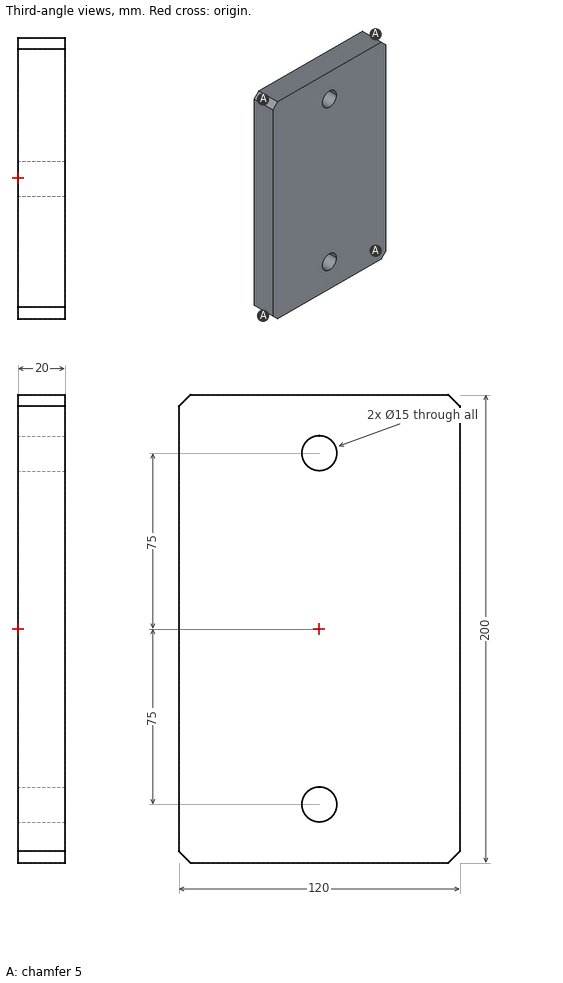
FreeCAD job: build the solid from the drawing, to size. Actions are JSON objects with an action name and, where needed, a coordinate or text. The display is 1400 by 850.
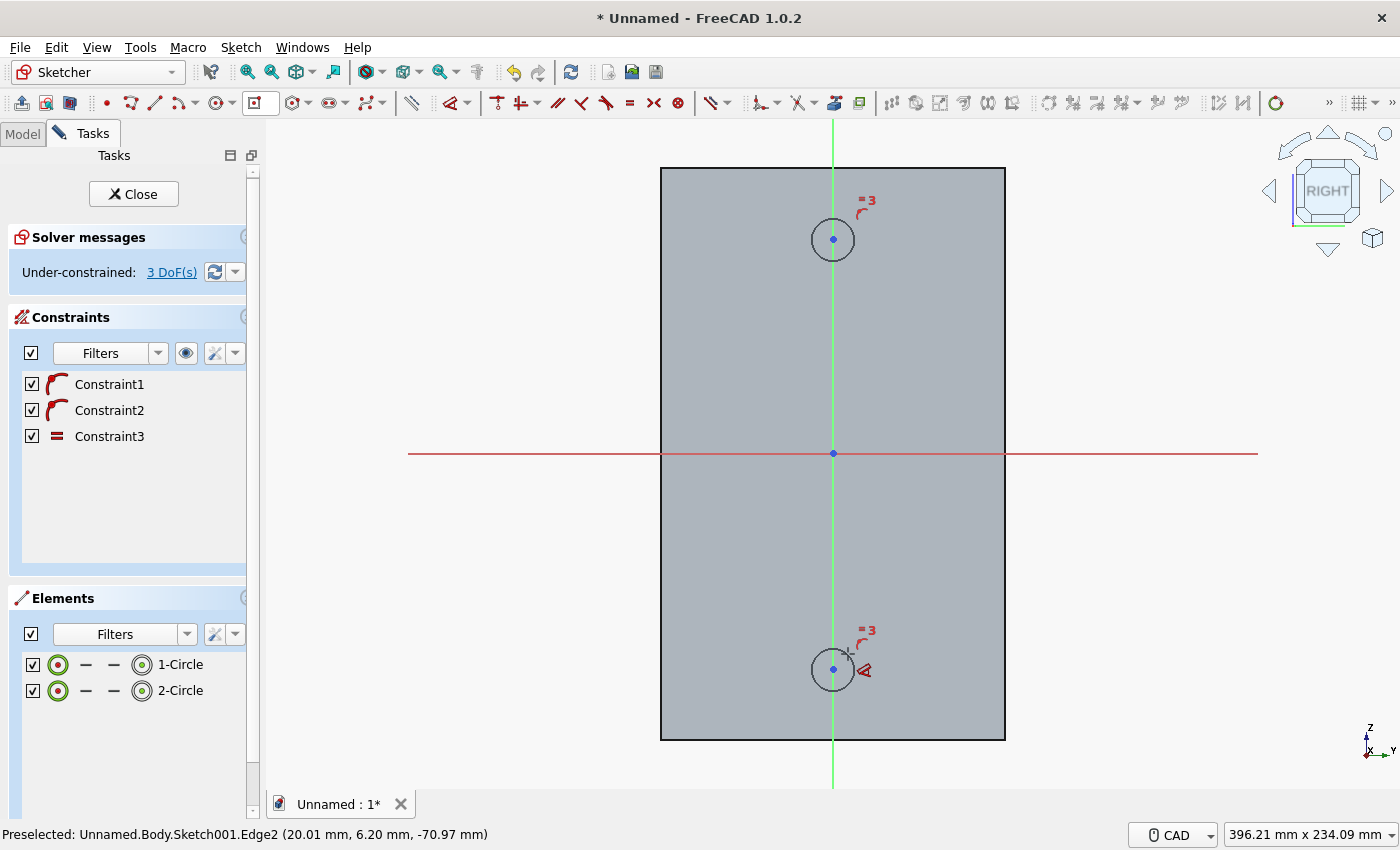
{"action": "left_click", "coordinate": [848, 225]}
{"action": "left_click", "coordinate": [871, 202]}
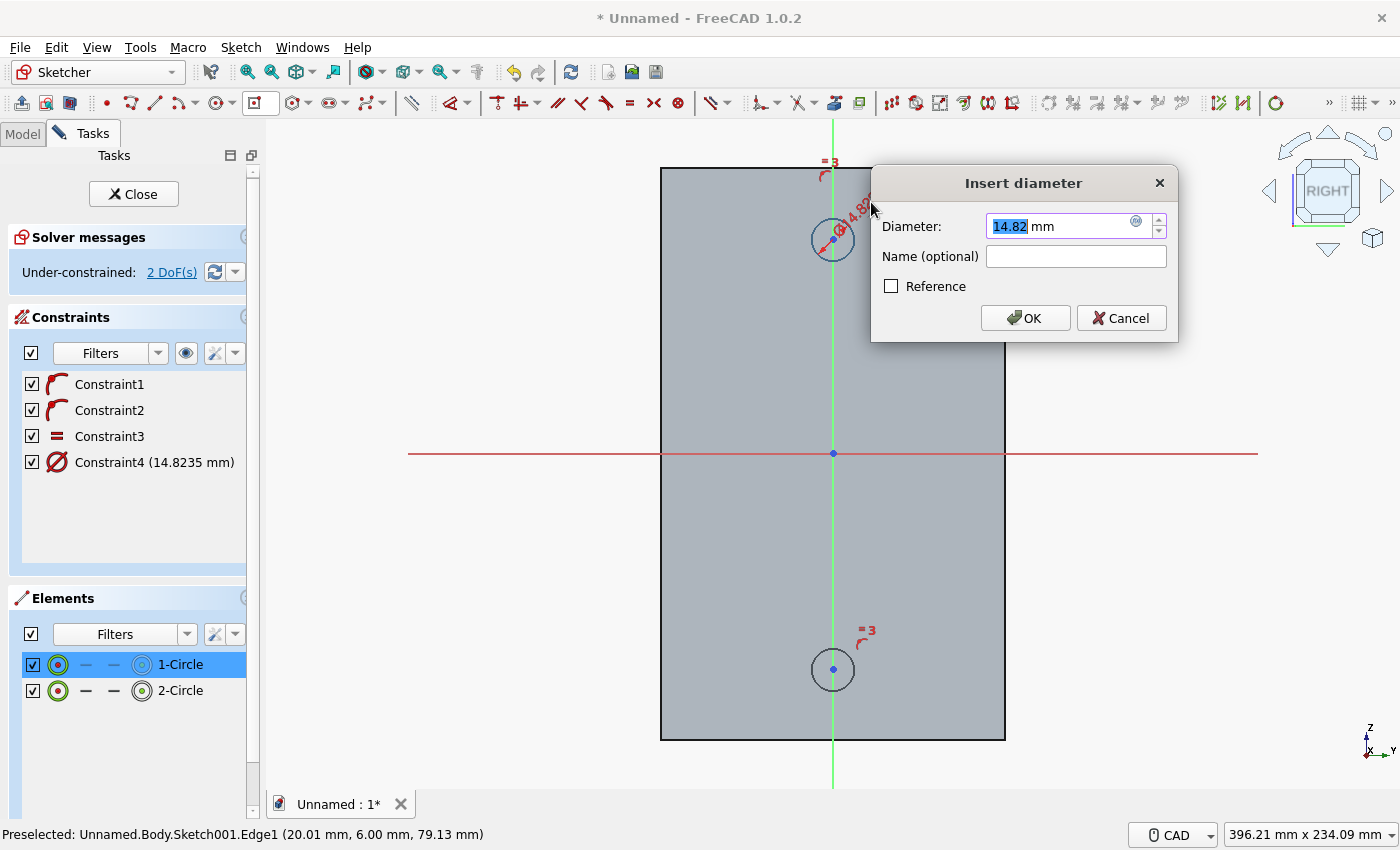
{"action": "type", "text": "15"}
{"action": "key", "text": "Return"}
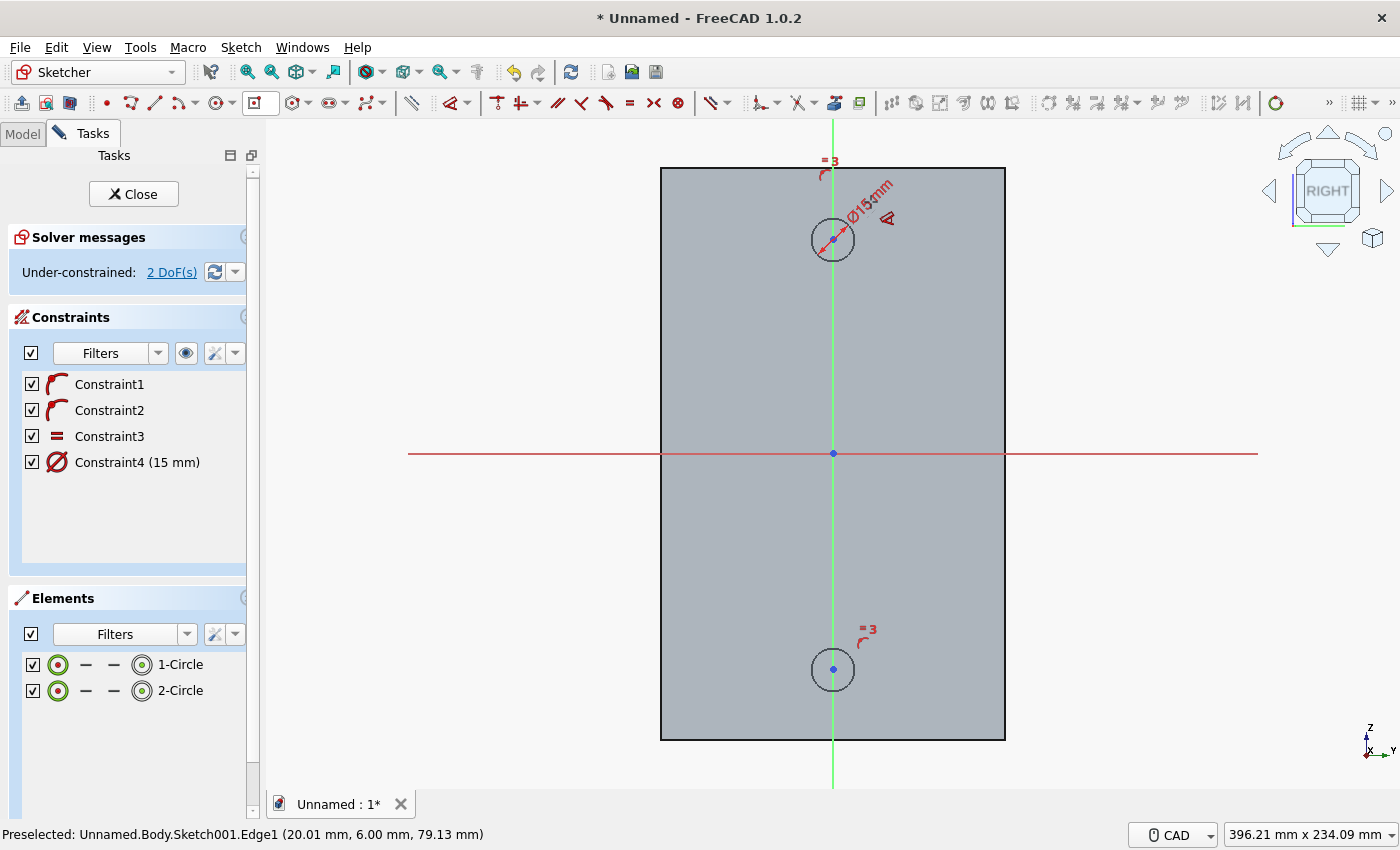
{"action": "left_click", "coordinate": [833, 240]}
{"action": "left_click", "coordinate": [867, 347]}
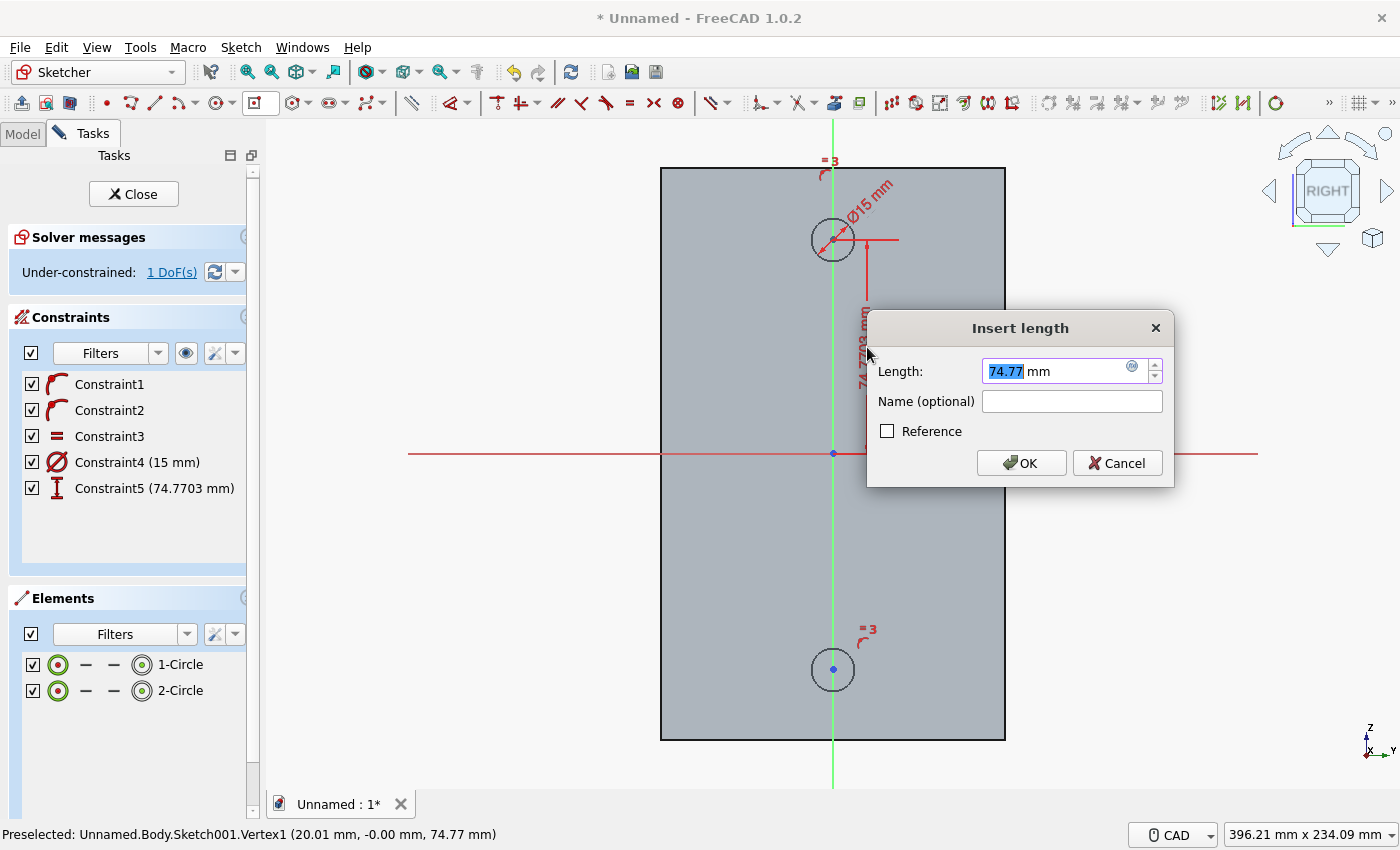
{"action": "type", "text": "75"}
{"action": "key", "text": "Return"}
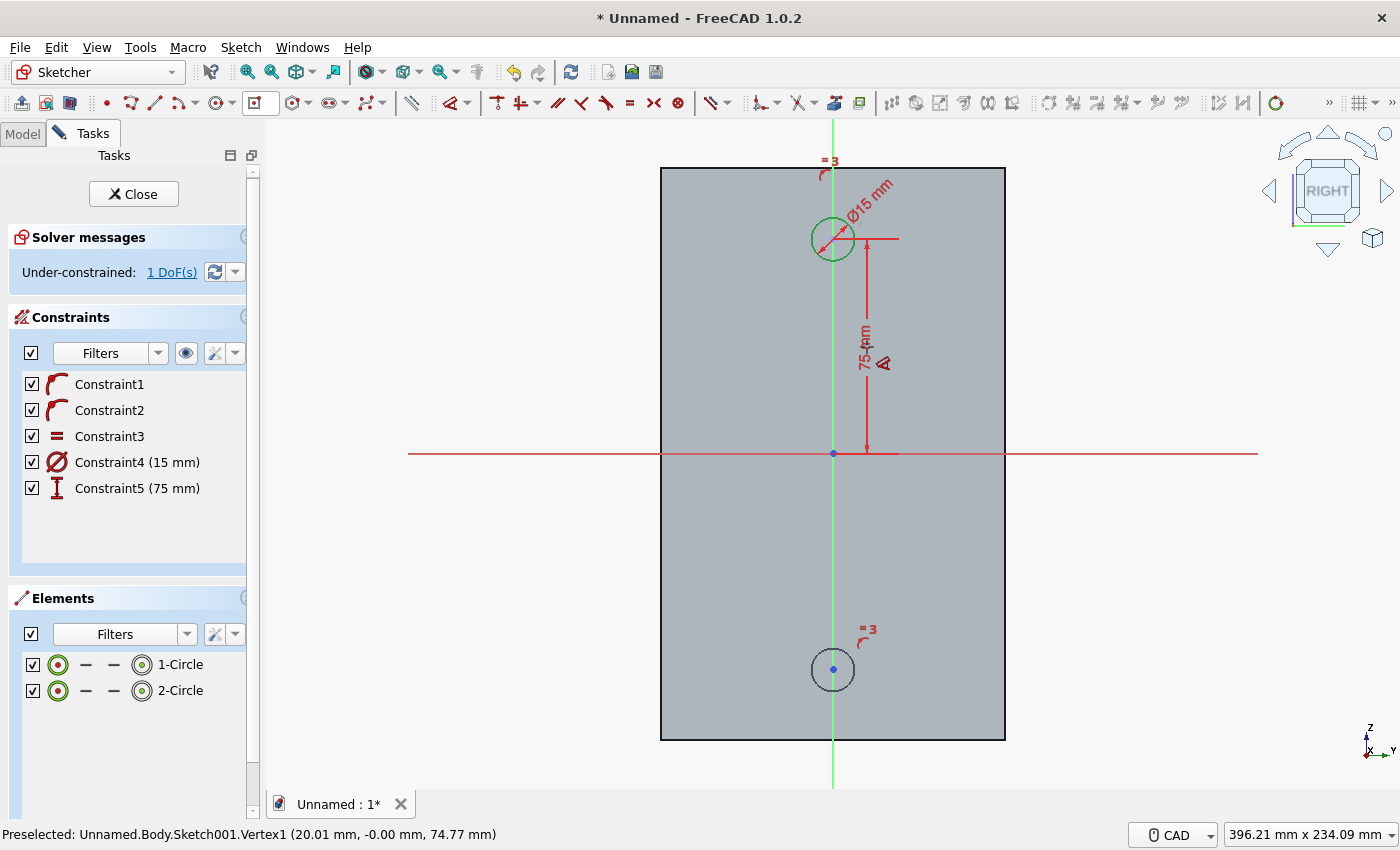
{"action": "left_click", "coordinate": [833, 670]}
{"action": "left_click", "coordinate": [867, 562]}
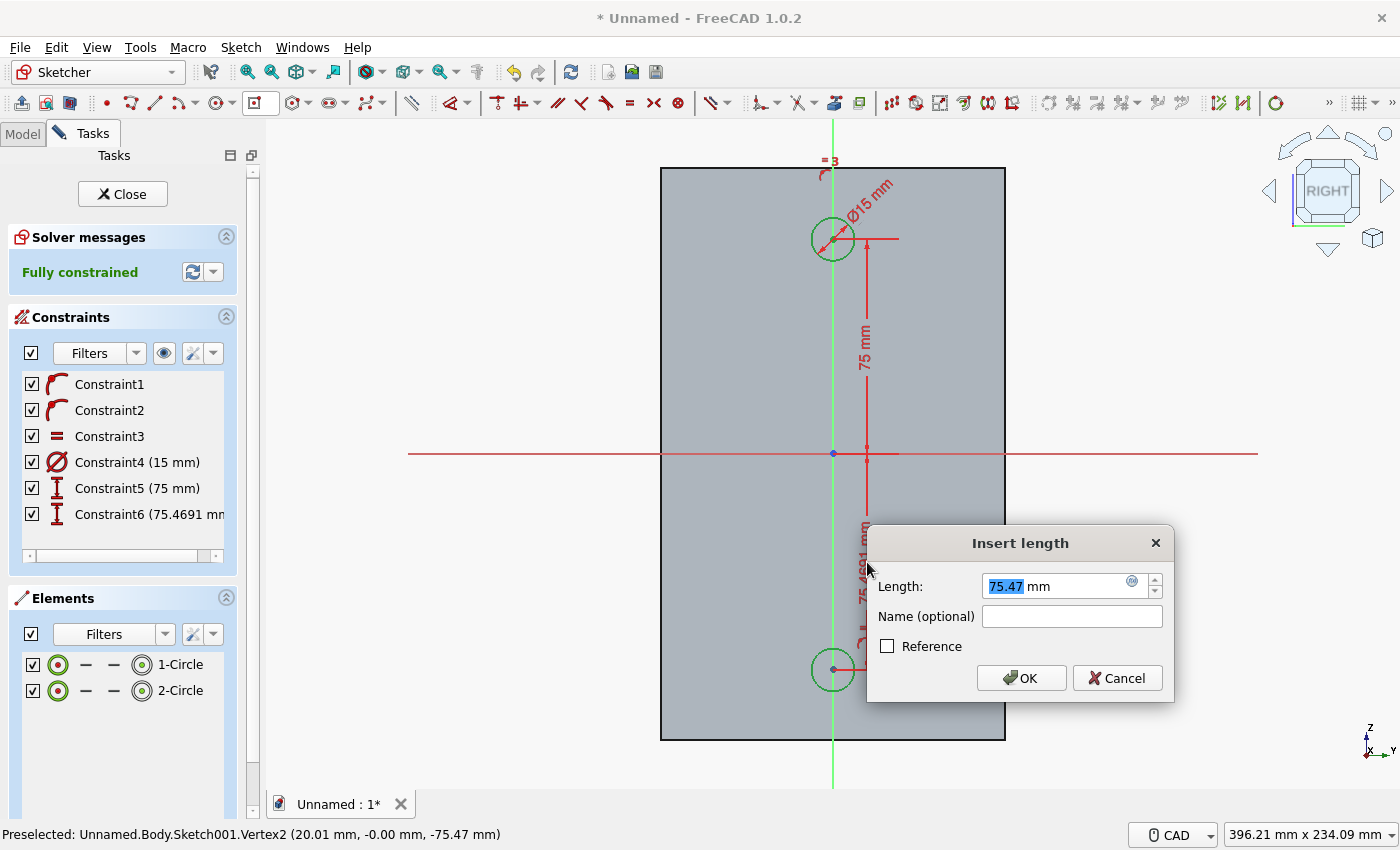
{"action": "type", "text": "75"}
{"action": "key", "text": "Return"}
{"action": "key", "text": "Escape"}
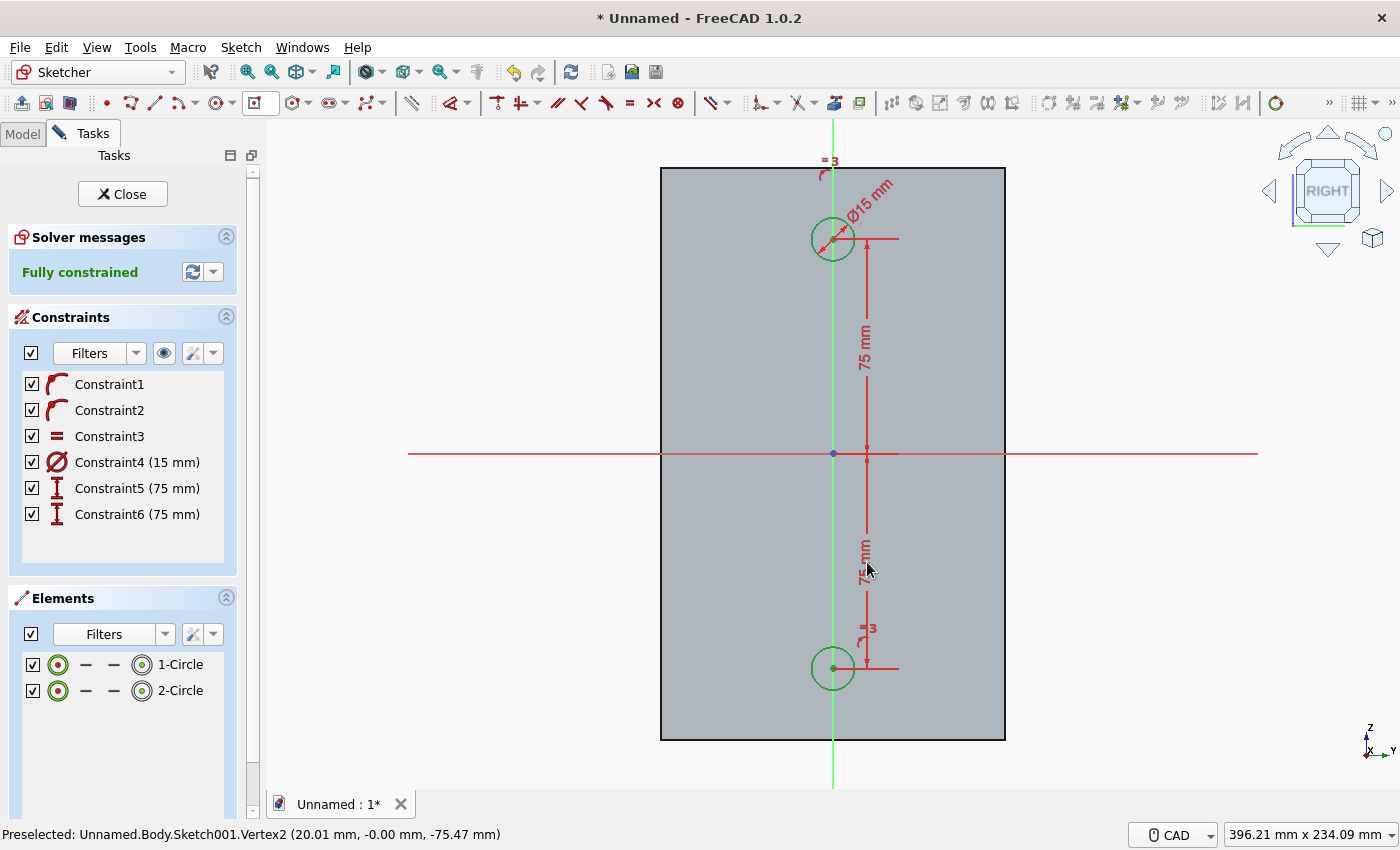
{"action": "left_click", "coordinate": [123, 194]}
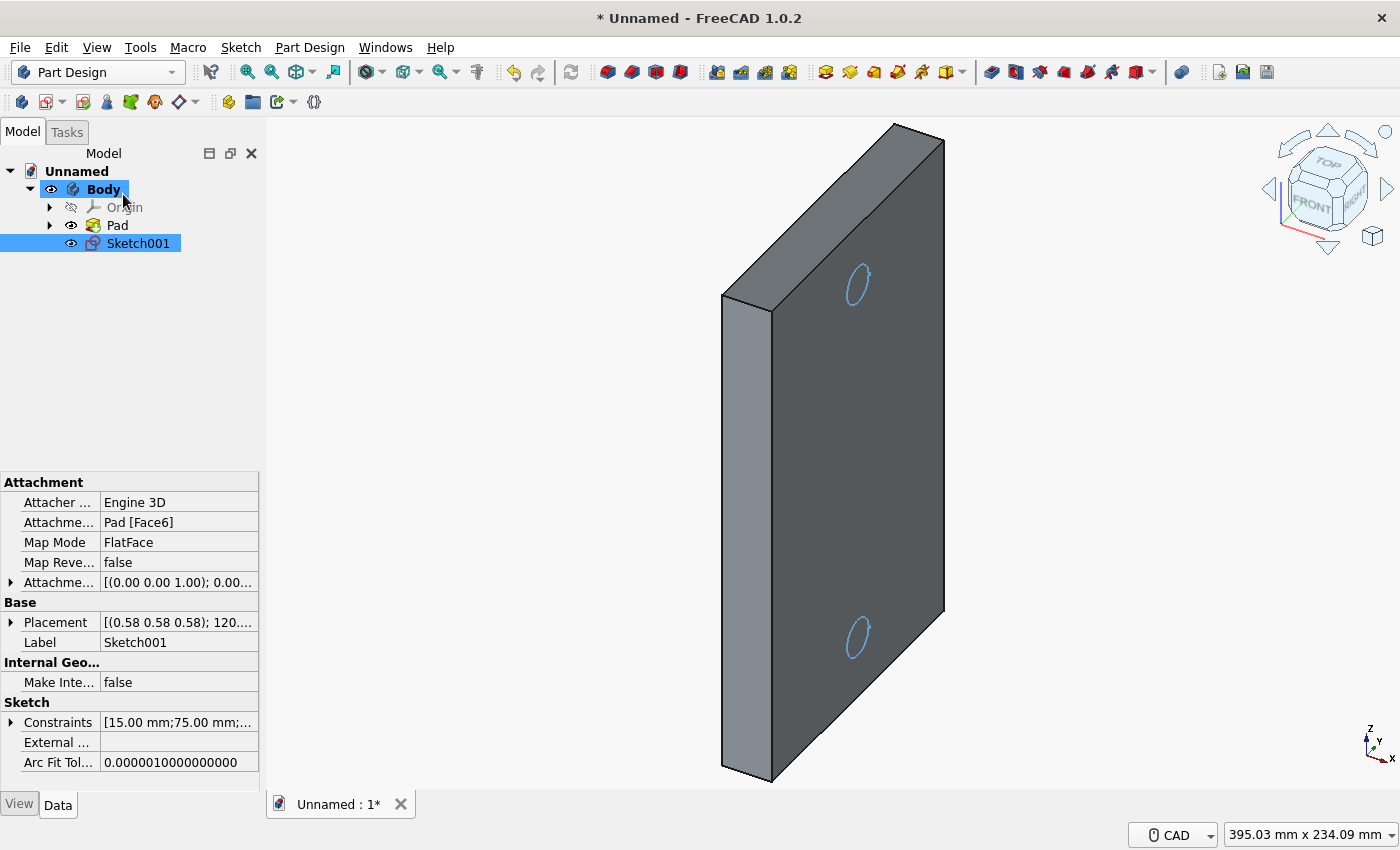
{"action": "left_click", "coordinate": [1016, 72]}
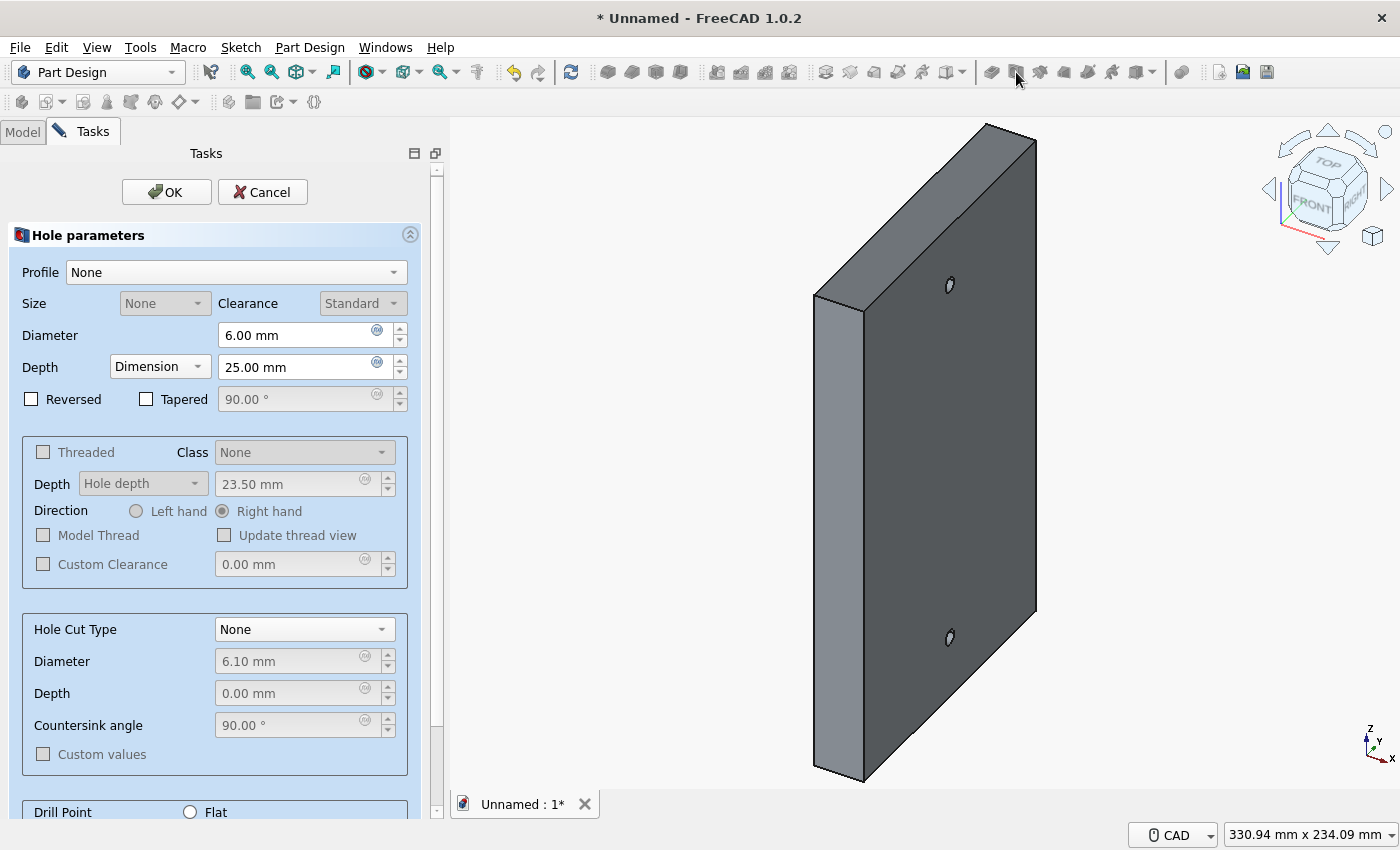
{"action": "triple_click", "coordinate": [305, 335]}